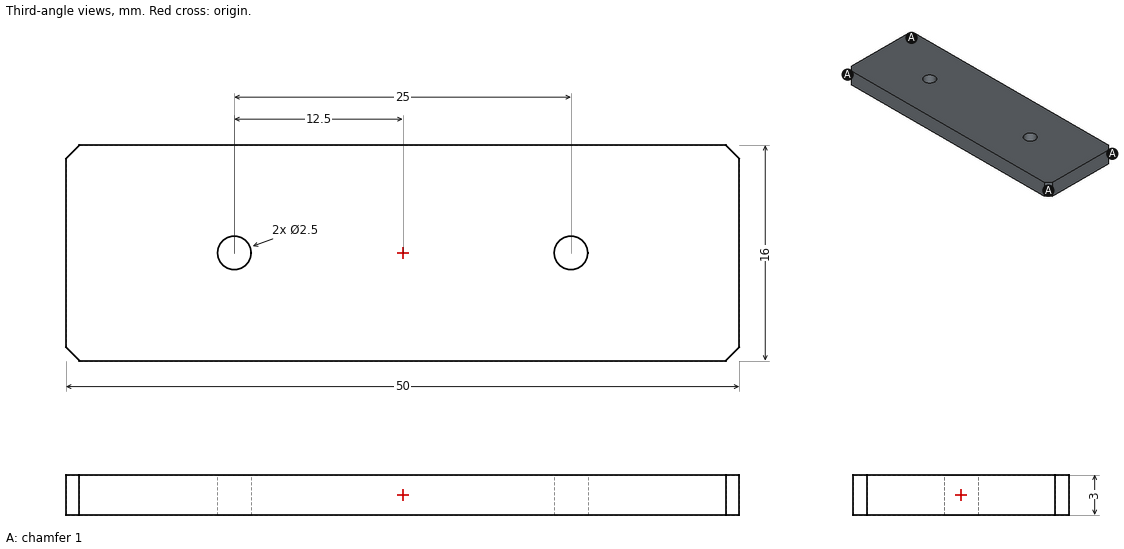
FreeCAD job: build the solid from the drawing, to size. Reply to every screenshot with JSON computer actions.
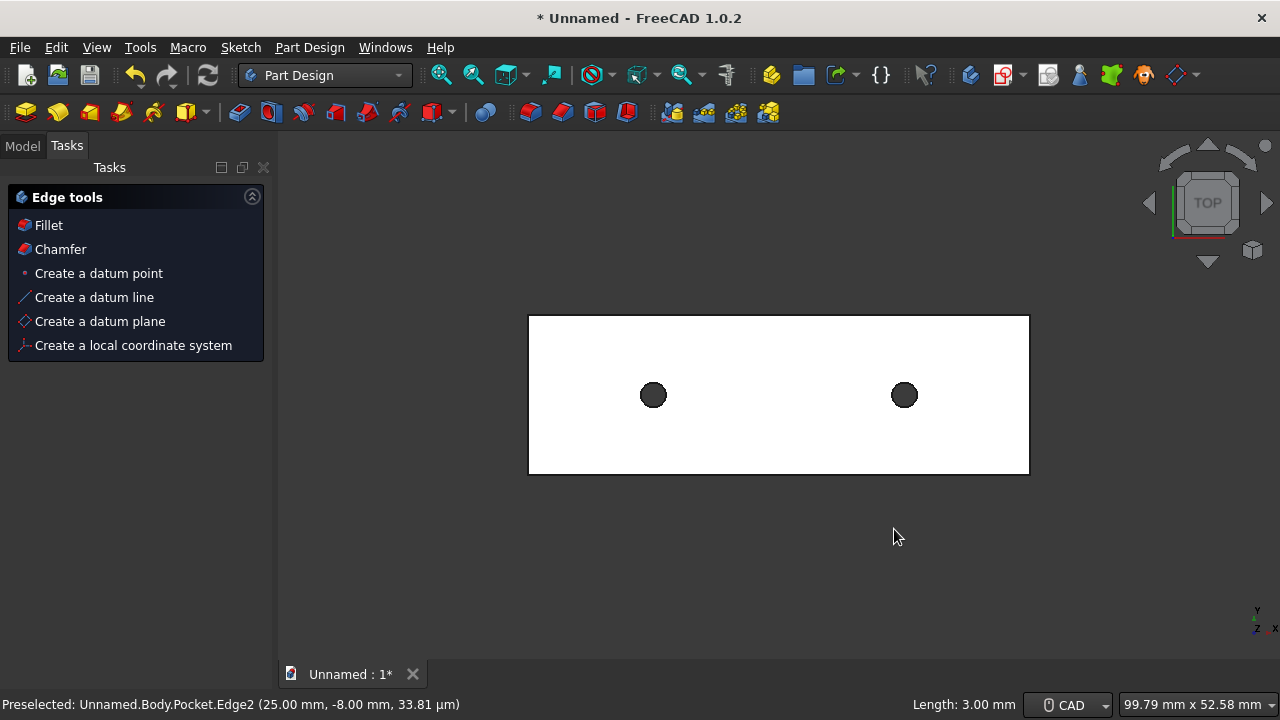
{"action": "key", "text": "1"}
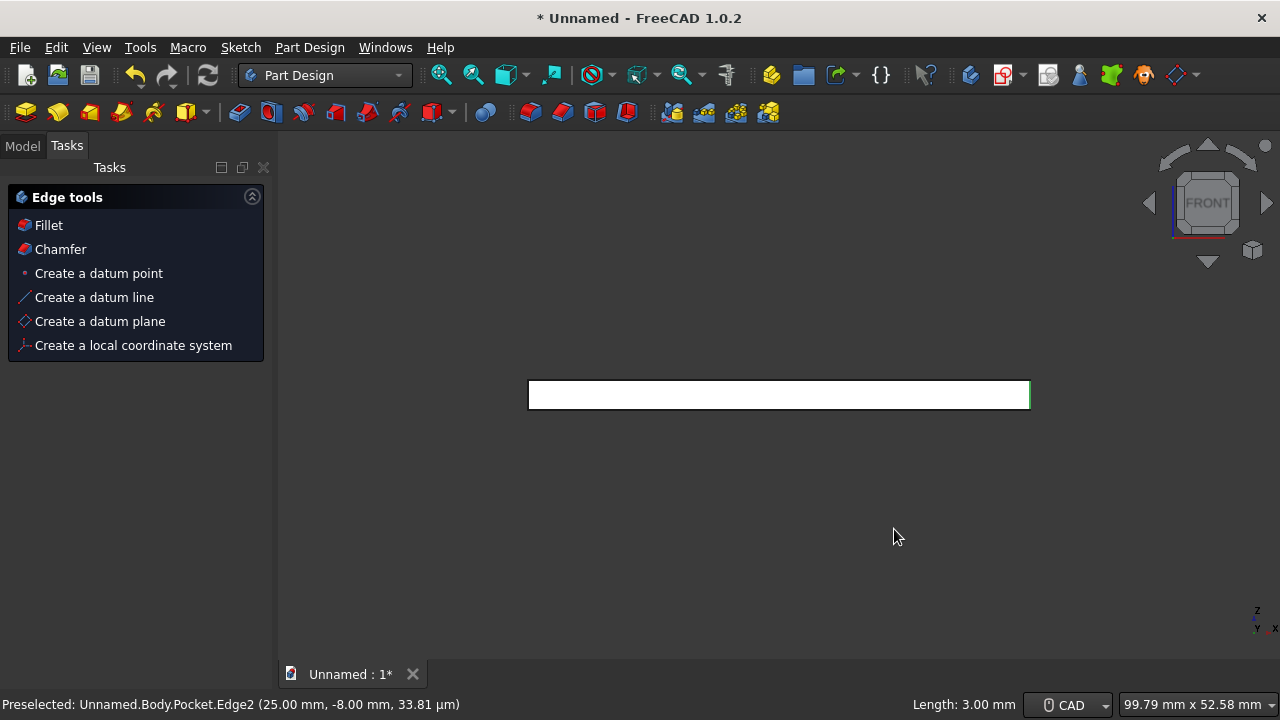
{"action": "left_click", "coordinate": [528, 394], "text": "ctrl"}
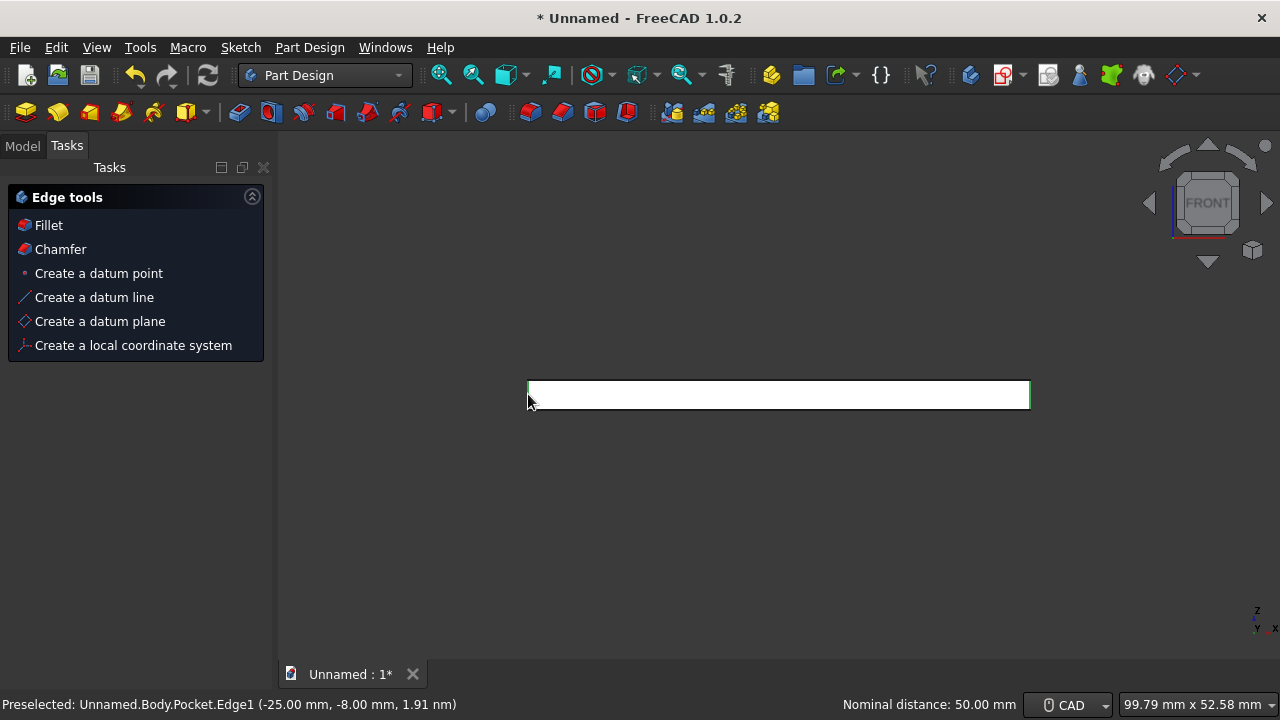
{"action": "key", "text": "3"}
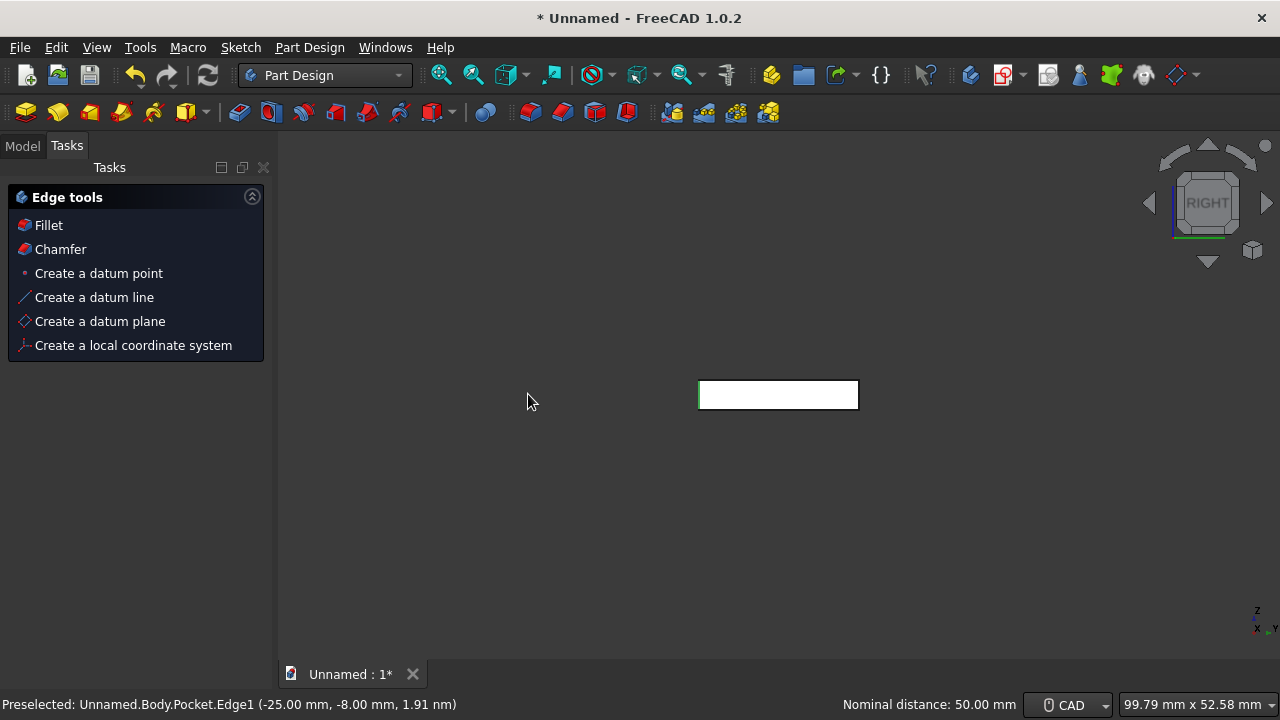
{"action": "left_click", "coordinate": [442, 76]}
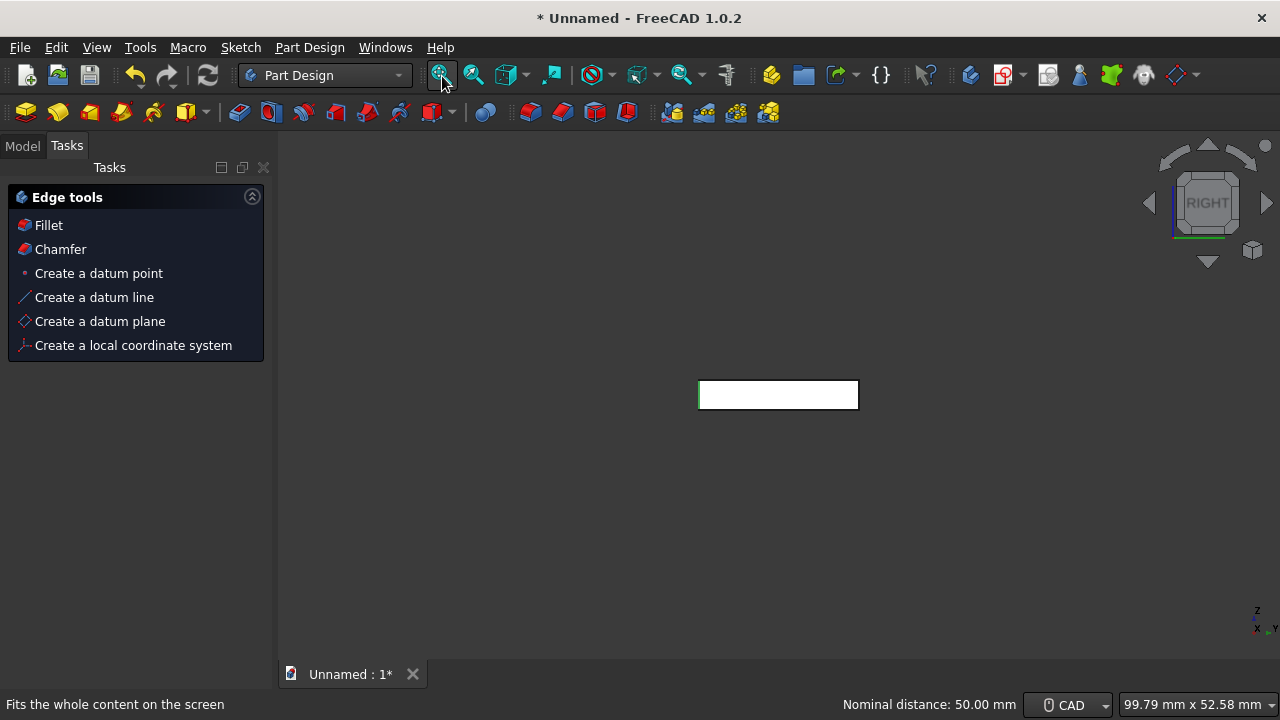
{"action": "left_click", "coordinate": [859, 394], "text": "ctrl"}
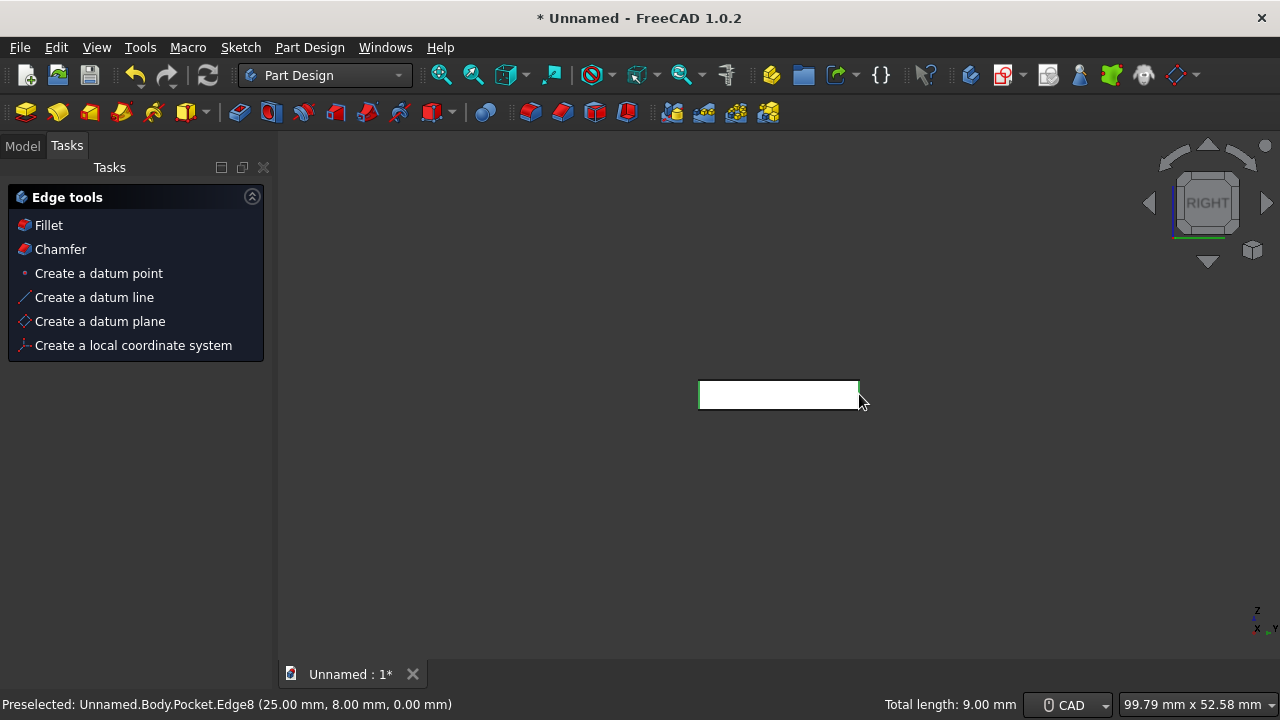
{"action": "key", "text": "5"}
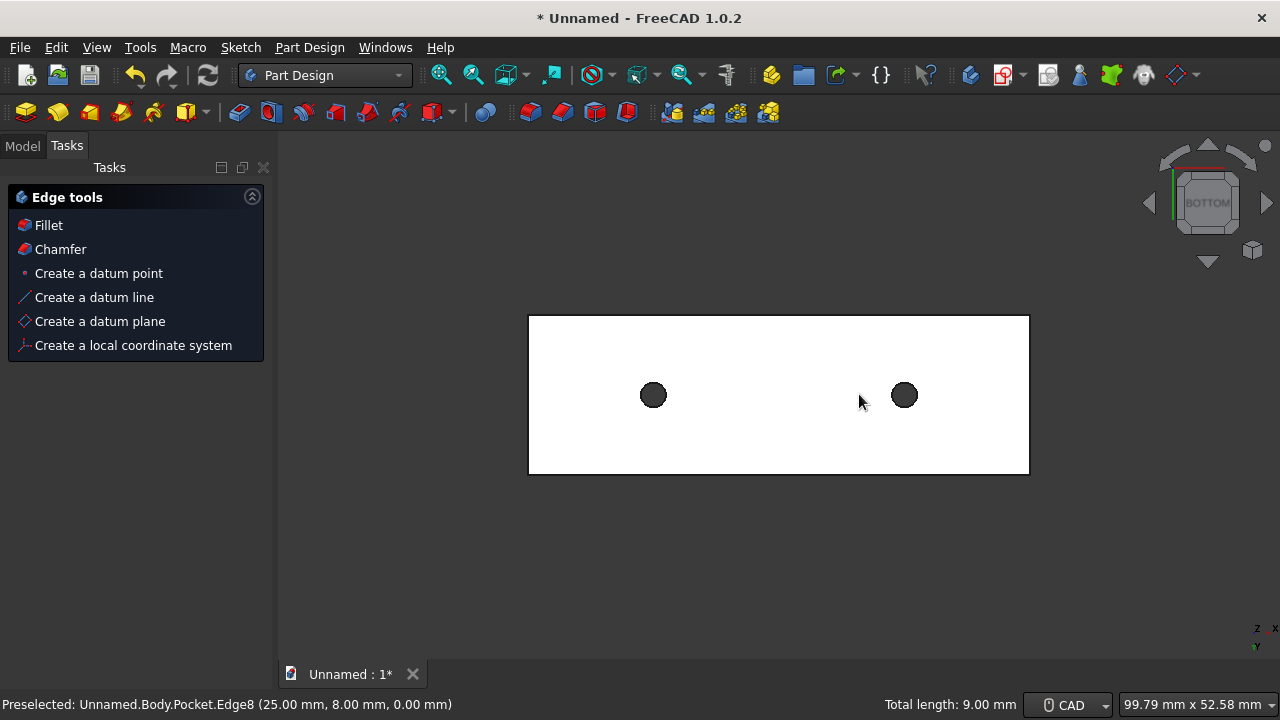
{"action": "key", "text": "4"}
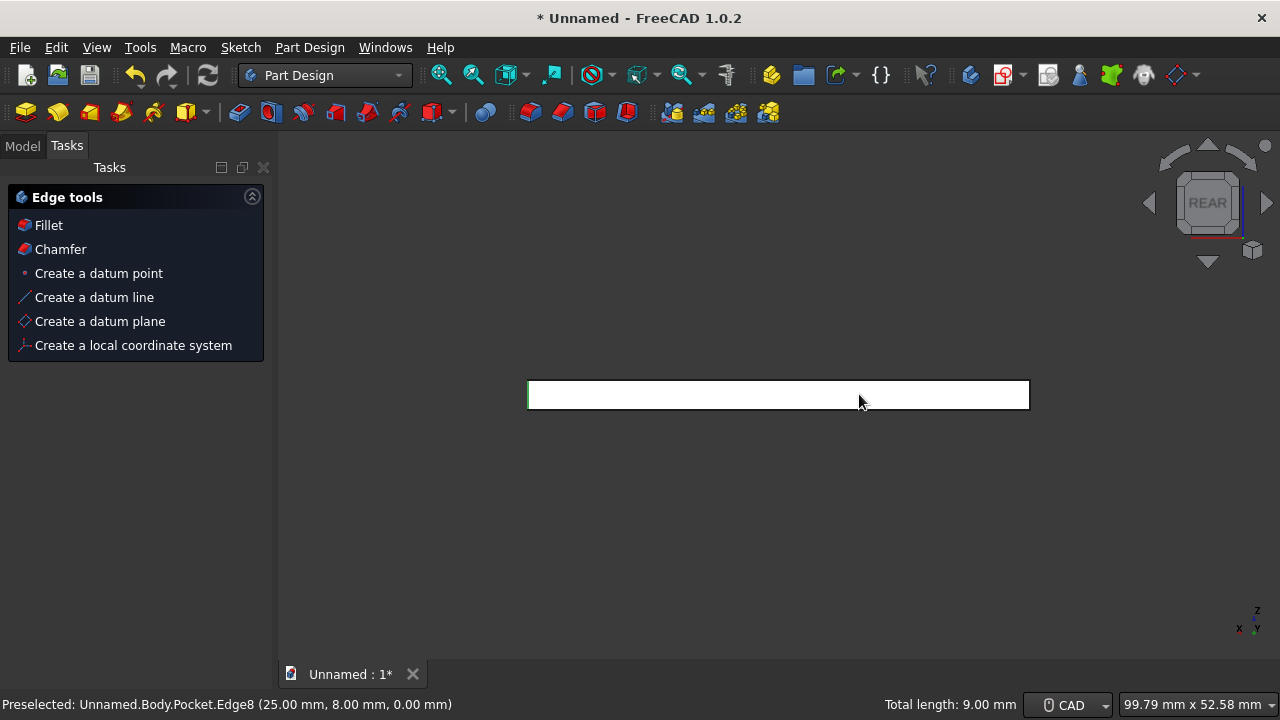
{"action": "left_click", "coordinate": [1030, 394], "text": "ctrl"}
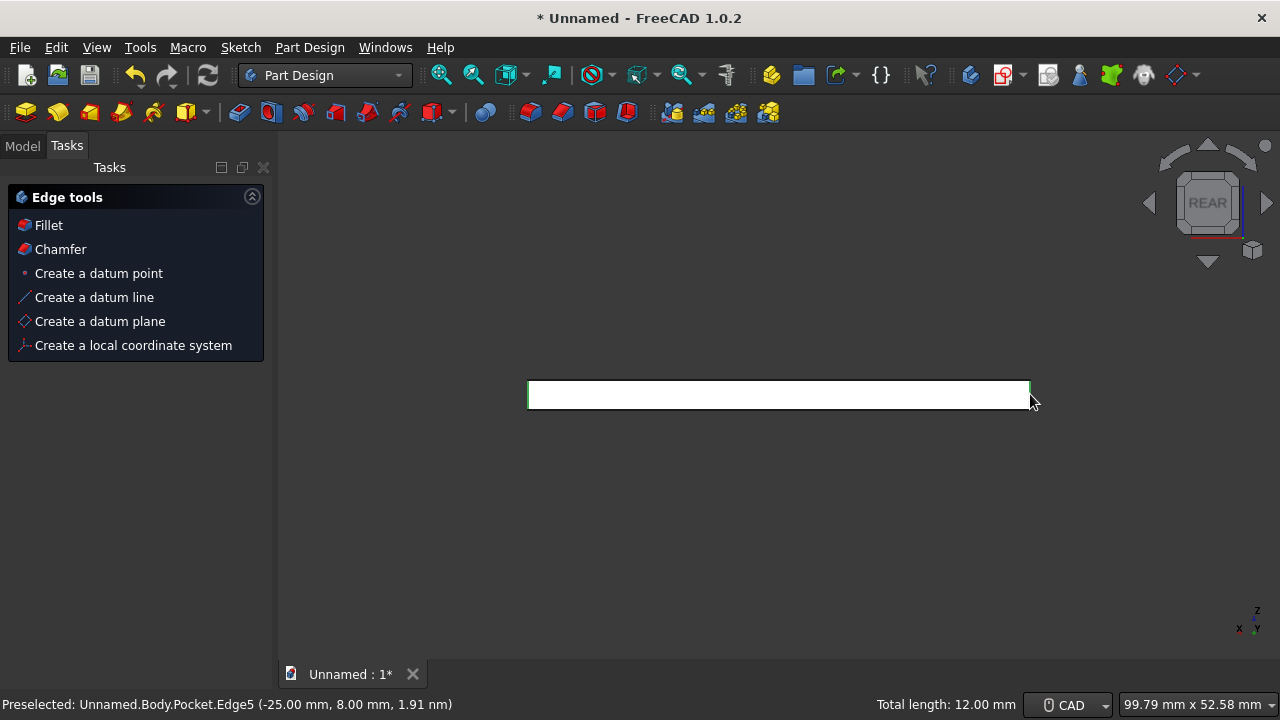
{"action": "left_click", "coordinate": [564, 112]}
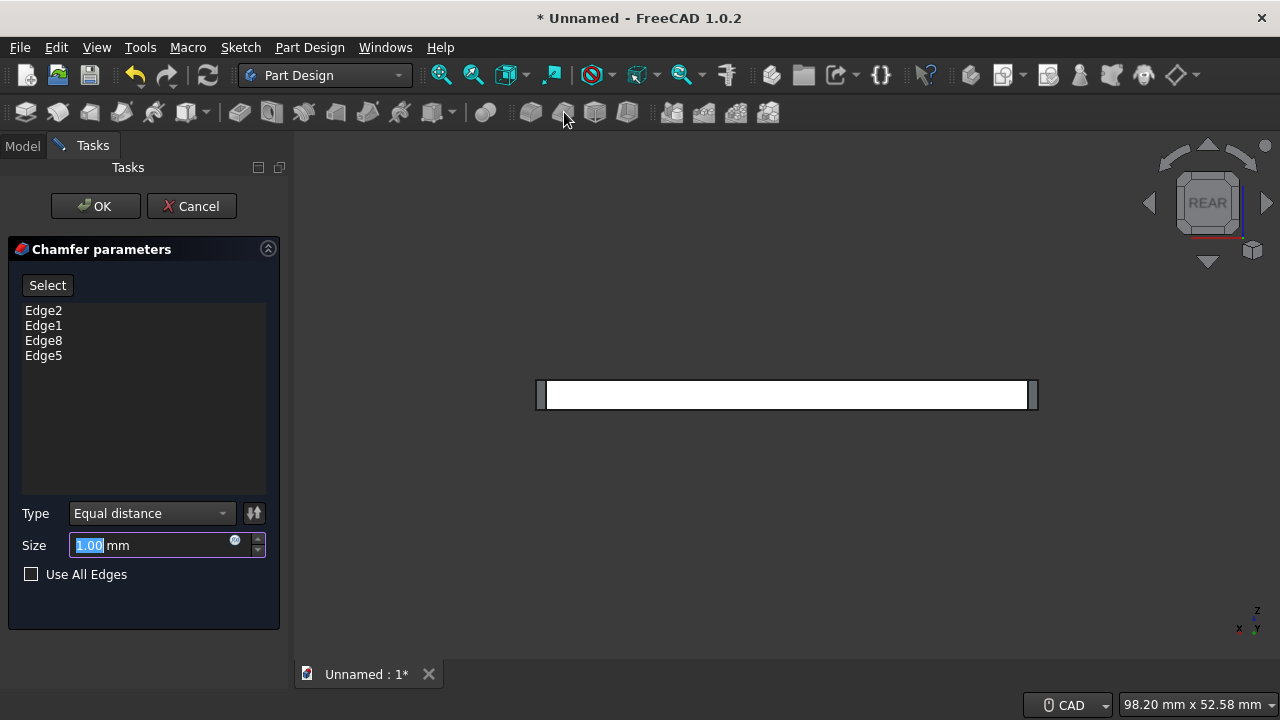
{"action": "type", "text": "1"}
{"action": "key", "text": "Tab"}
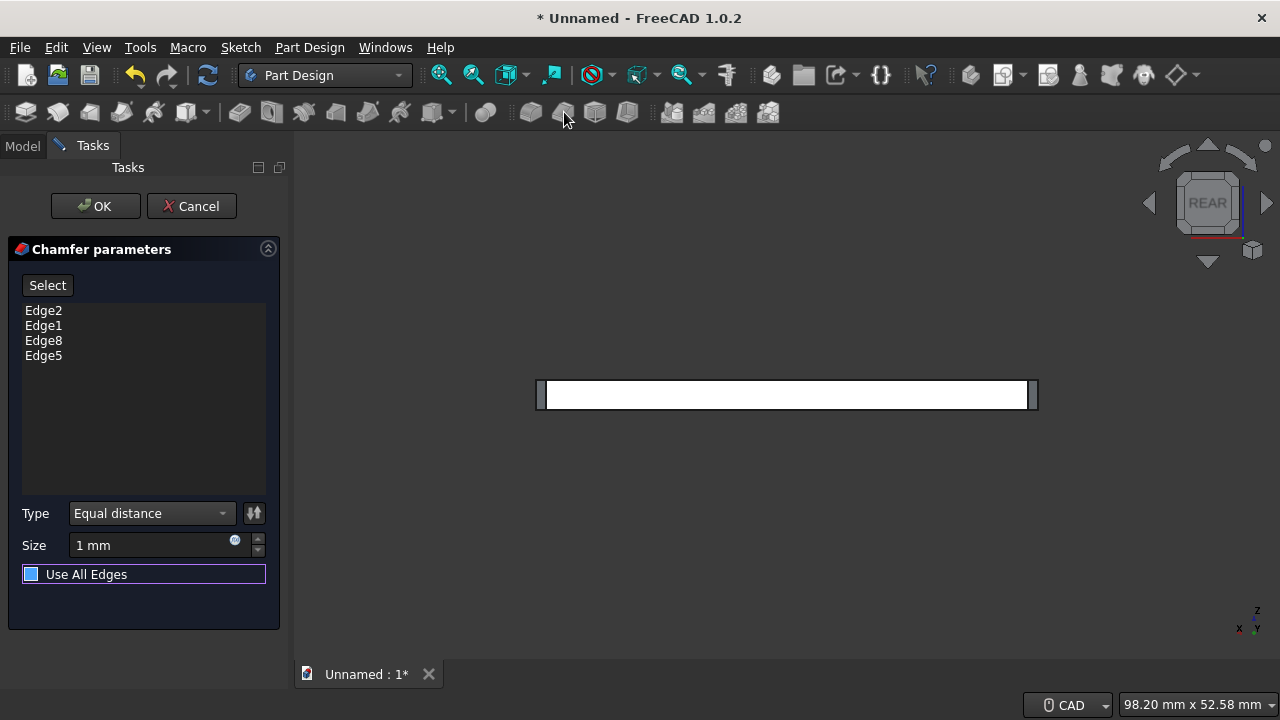
{"action": "left_click", "coordinate": [96, 206]}